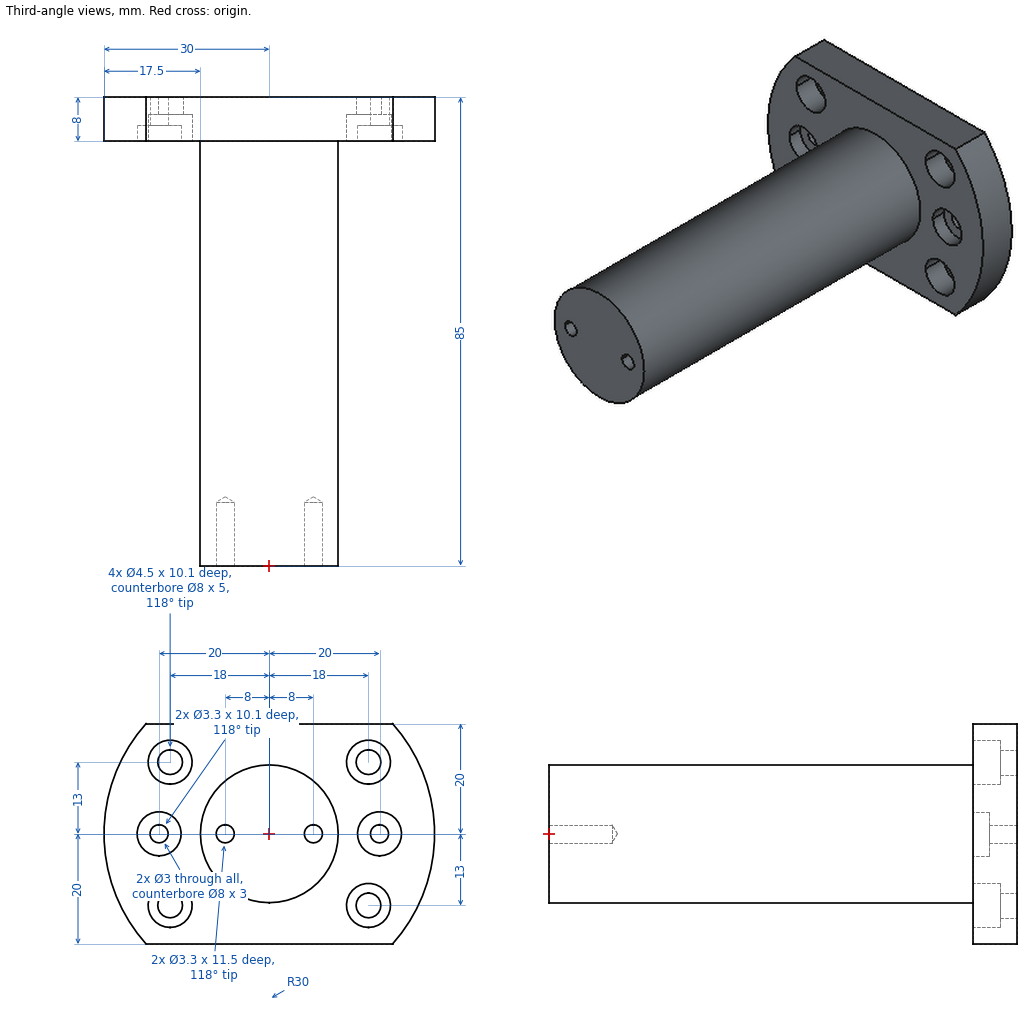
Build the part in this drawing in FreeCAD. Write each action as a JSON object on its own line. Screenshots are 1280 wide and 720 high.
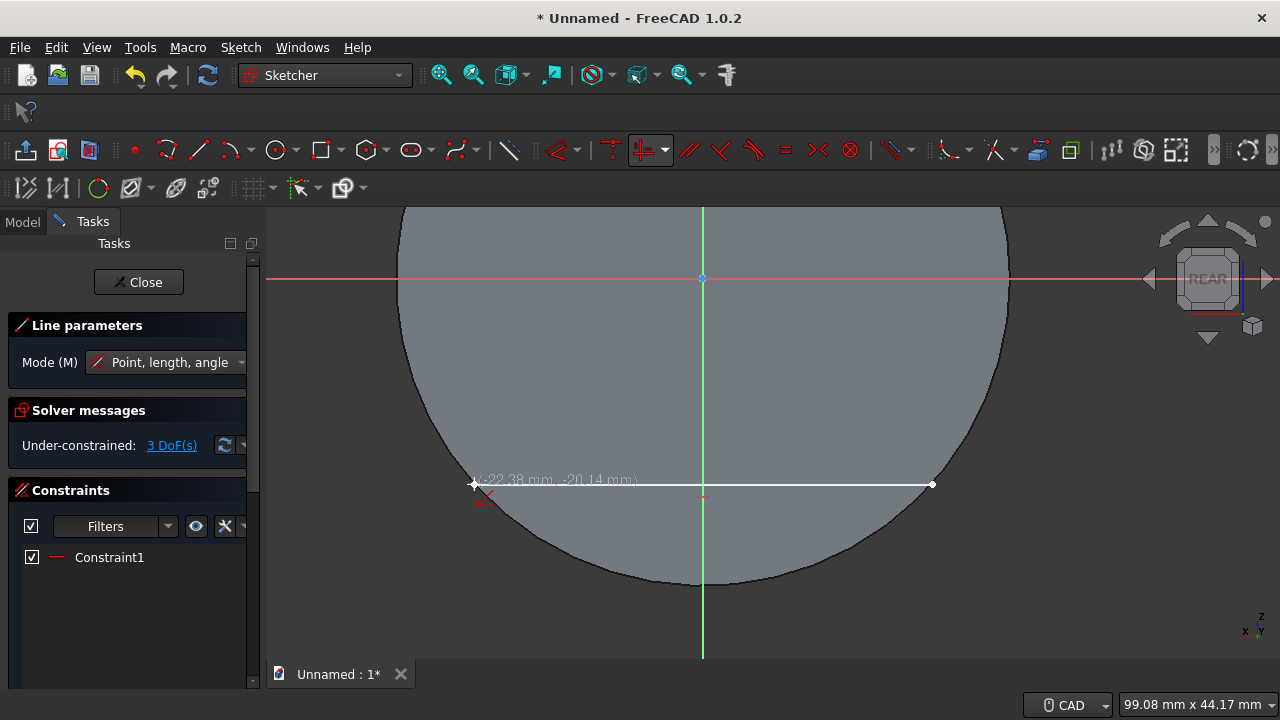
{"action": "left_click", "coordinate": [254, 150]}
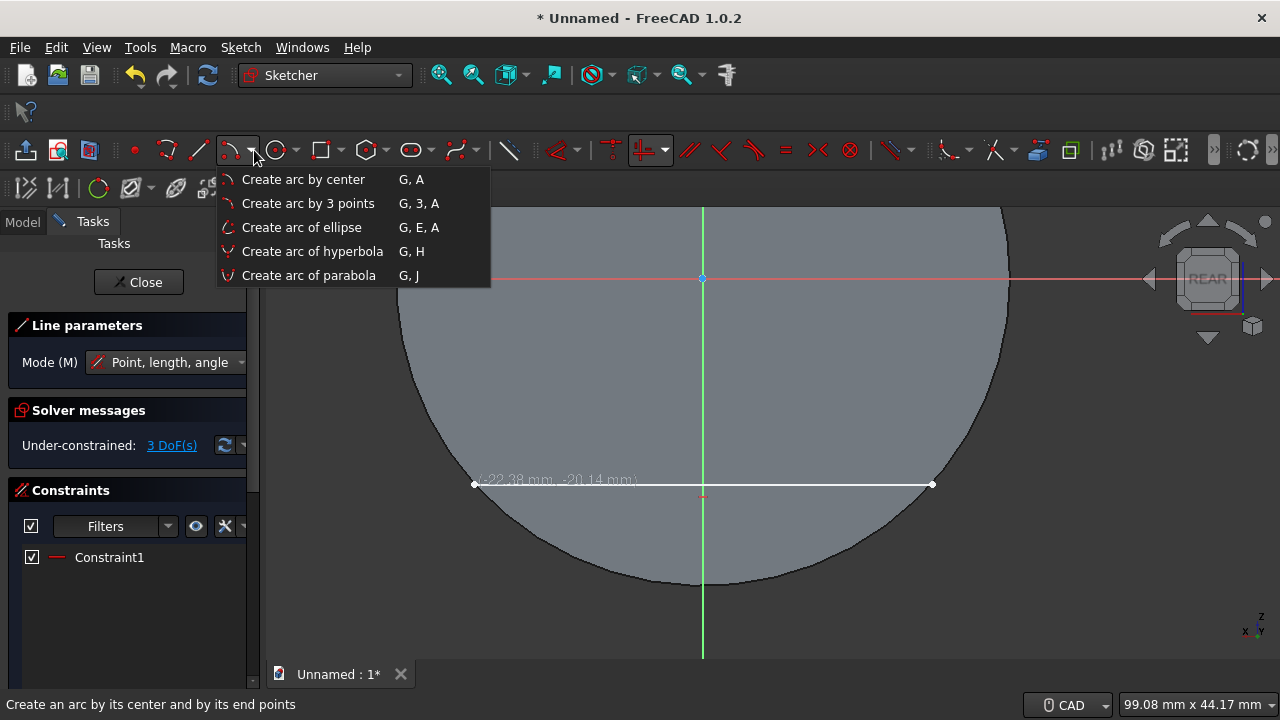
{"action": "left_click", "coordinate": [354, 203]}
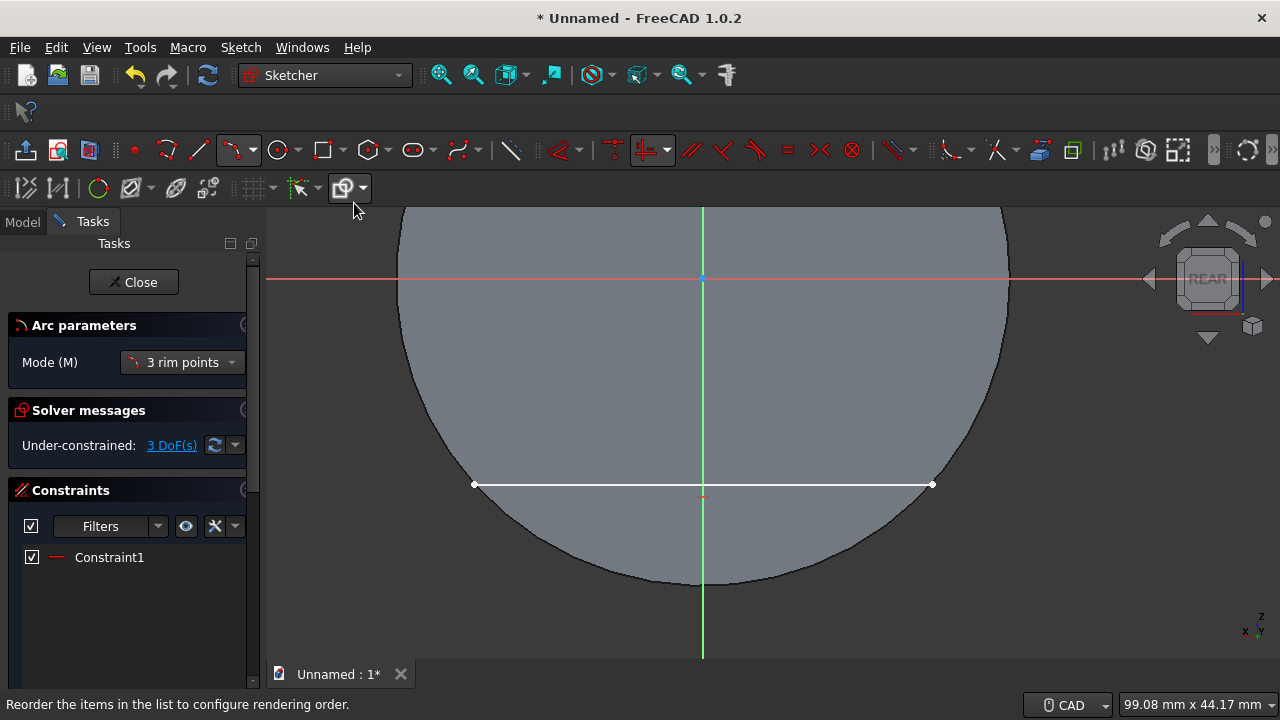
{"action": "left_click", "coordinate": [474, 485]}
{"action": "left_click", "coordinate": [932, 485]}
{"action": "left_click", "coordinate": [652, 582]}
{"action": "key", "text": "Escape"}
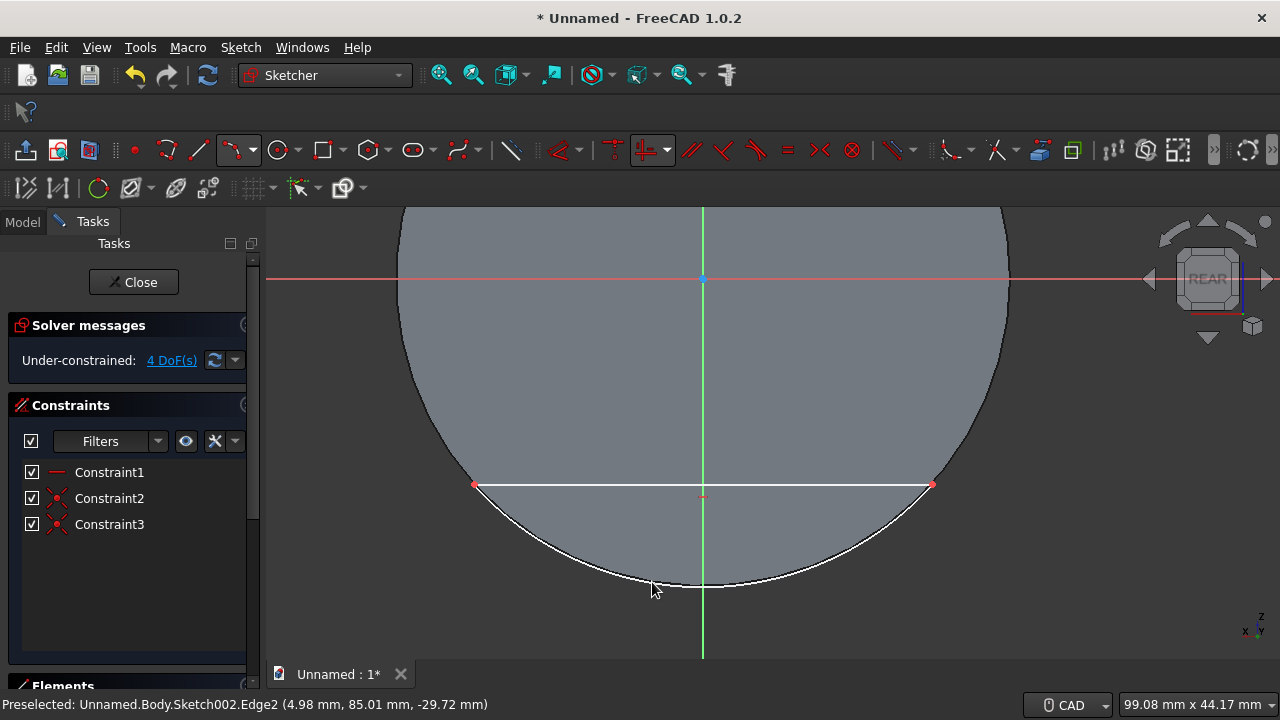
{"action": "left_click_drag", "start_coordinate": [693, 269], "coordinate": [713, 290]}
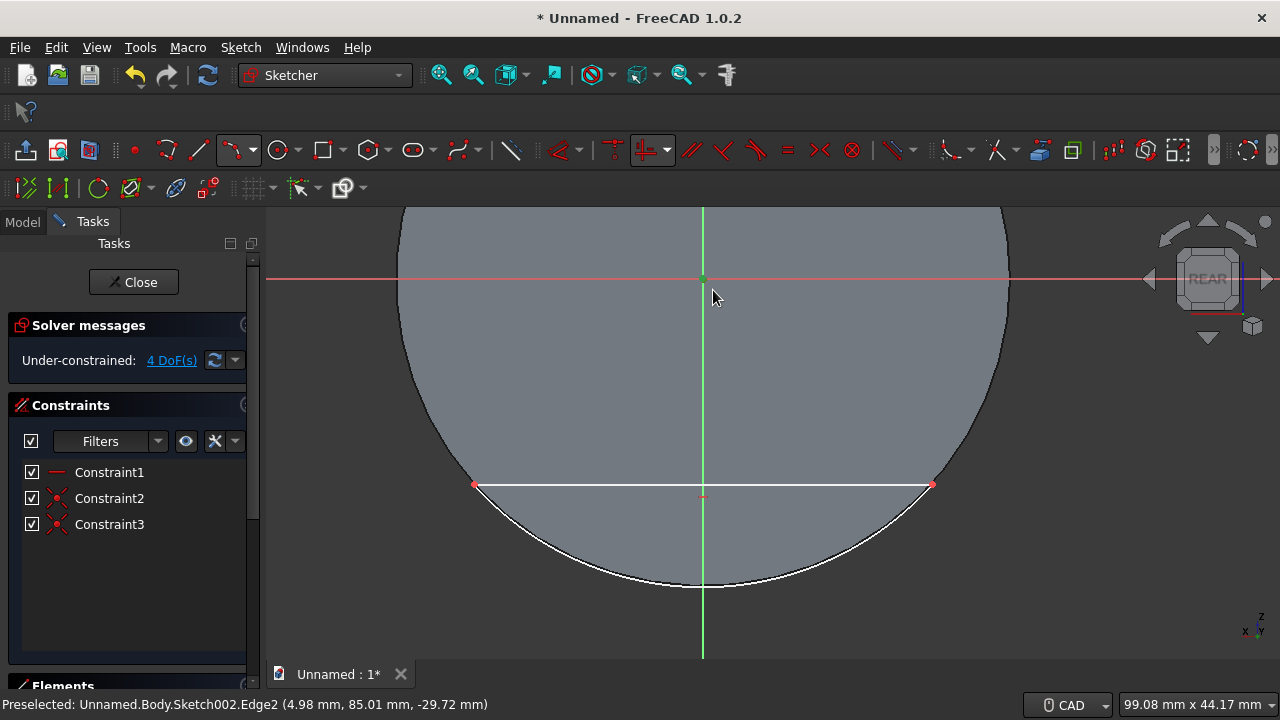
{"action": "left_click", "coordinate": [614, 150]}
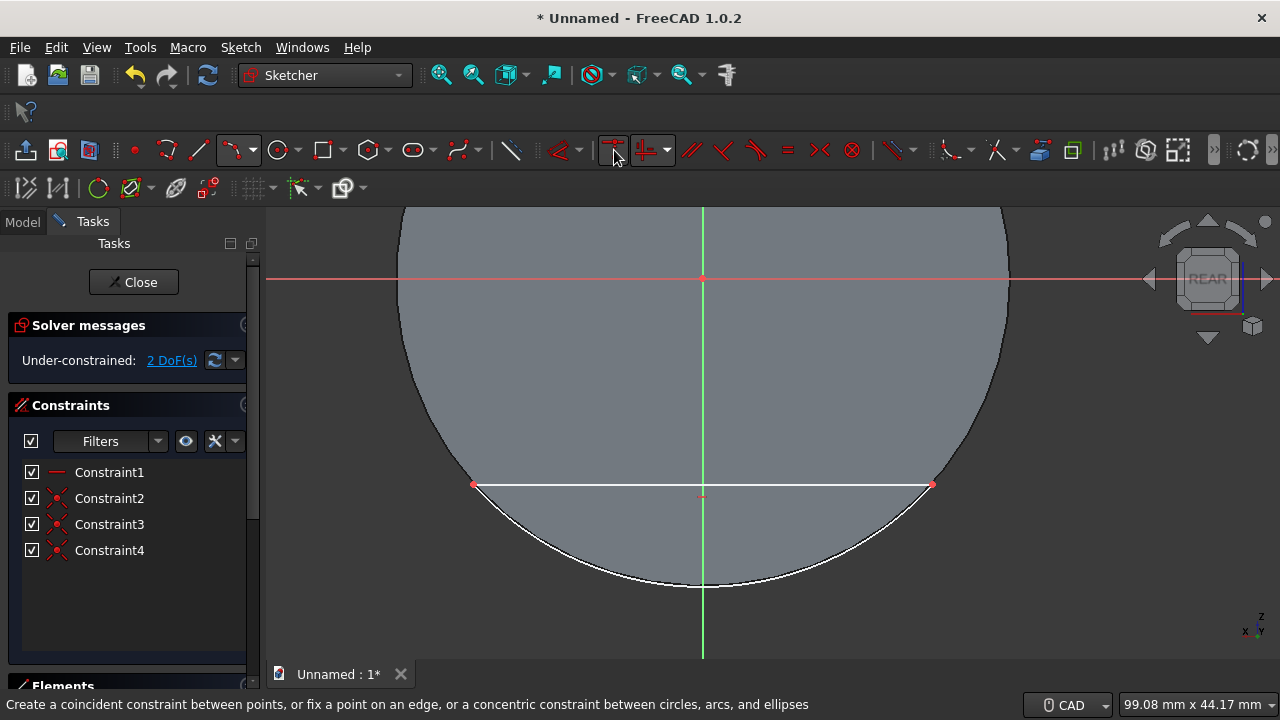
{"action": "left_click", "coordinate": [558, 150]}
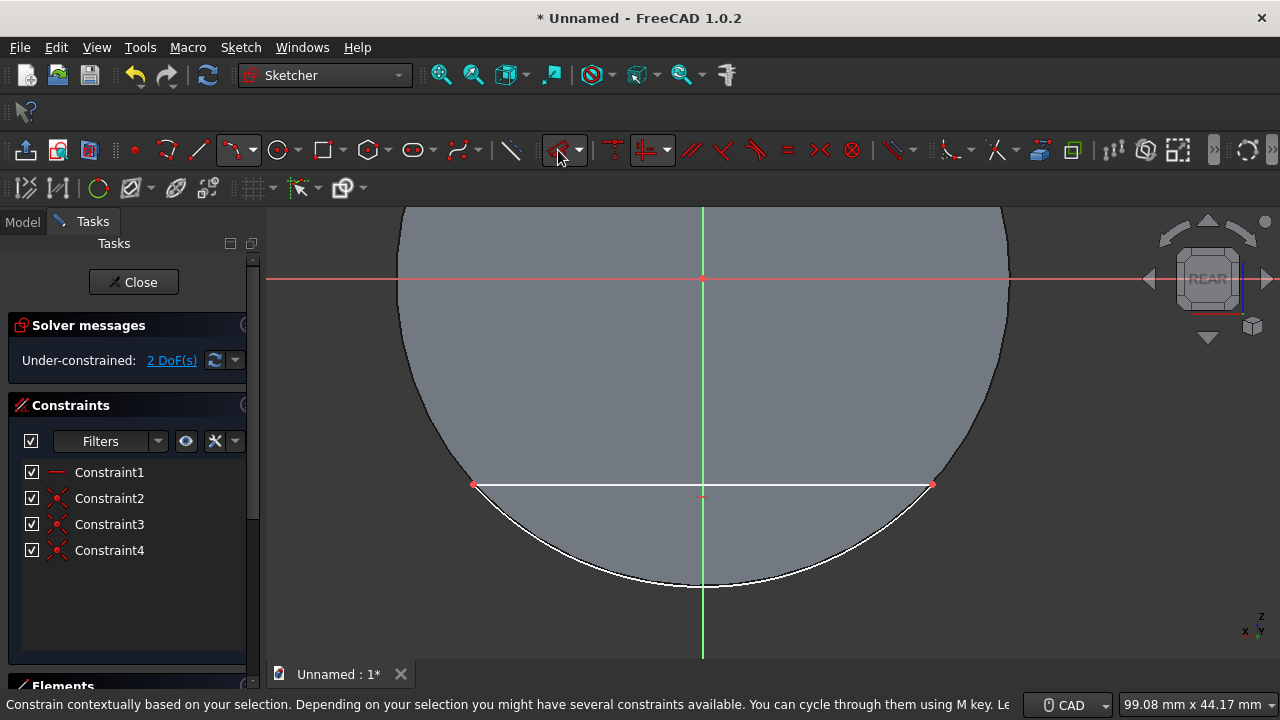
{"action": "left_click", "coordinate": [602, 570]}
{"action": "left_click", "coordinate": [592, 600]}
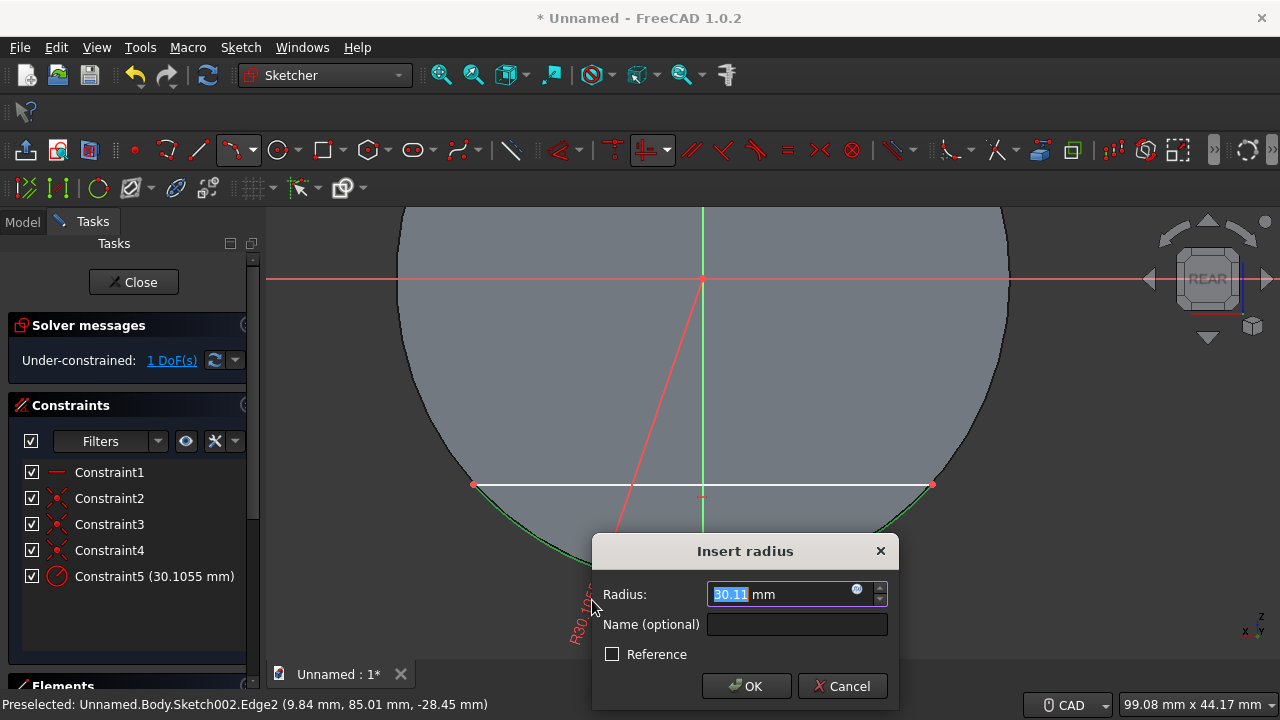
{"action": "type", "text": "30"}
{"action": "key", "text": "Return"}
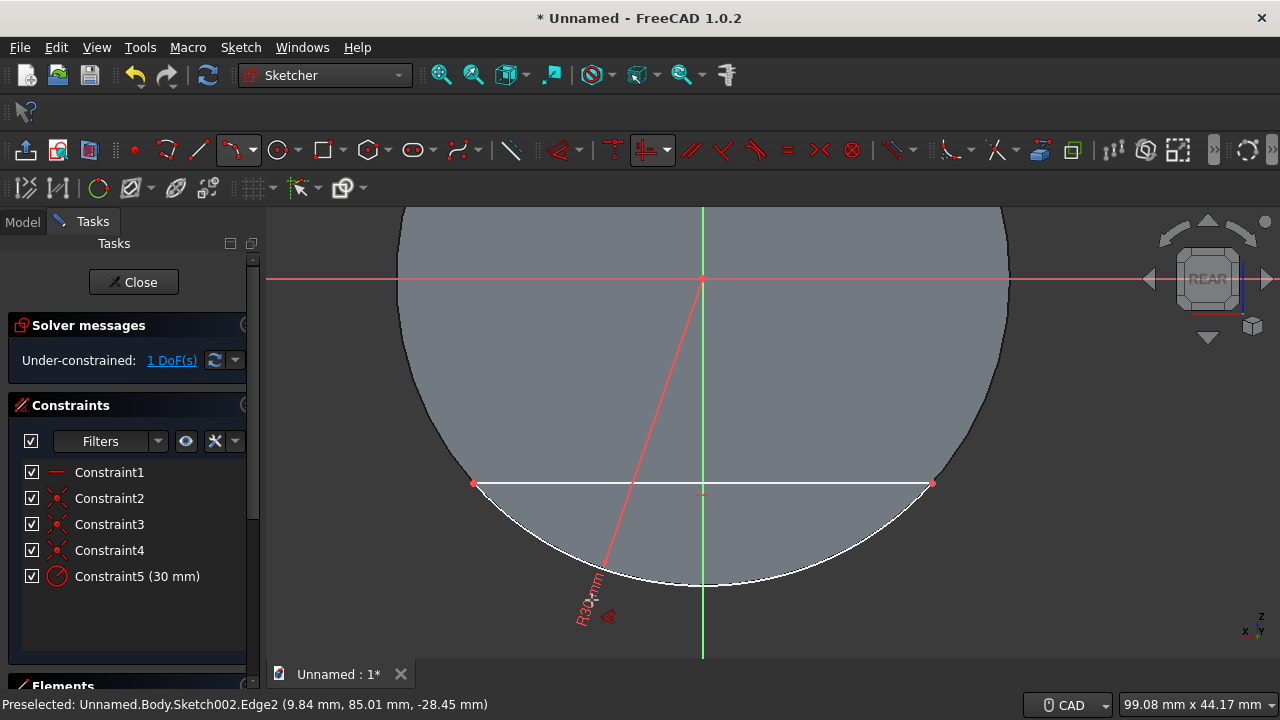
{"action": "left_click", "coordinate": [932, 483]}
{"action": "left_click", "coordinate": [966, 381]}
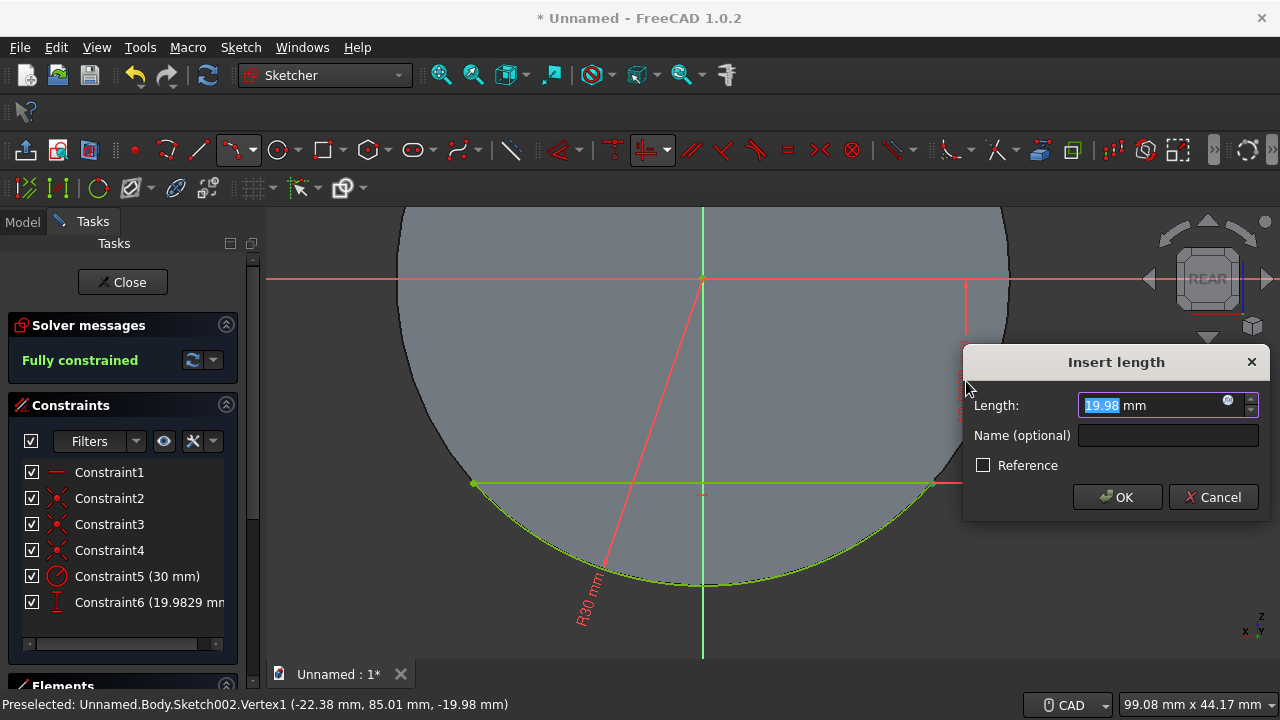
{"action": "type", "text": "20"}
{"action": "key", "text": "Return"}
{"action": "key", "text": "Escape"}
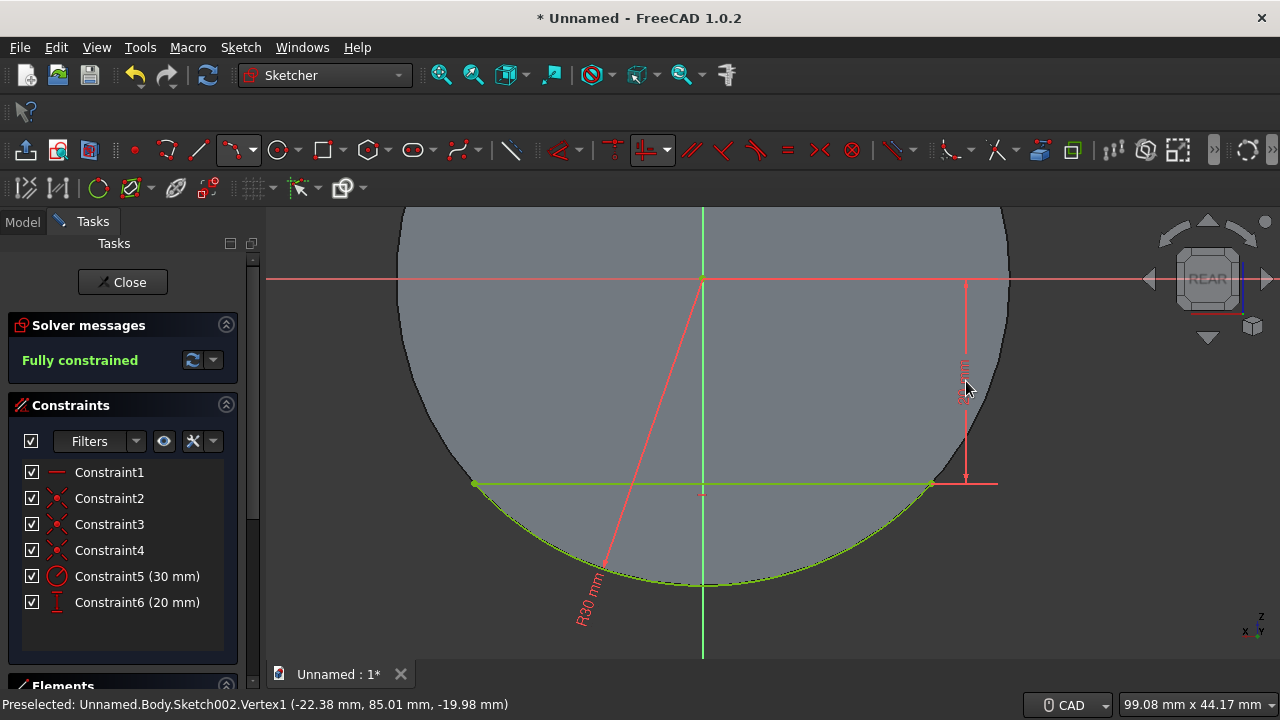
{"action": "left_click", "coordinate": [123, 282]}